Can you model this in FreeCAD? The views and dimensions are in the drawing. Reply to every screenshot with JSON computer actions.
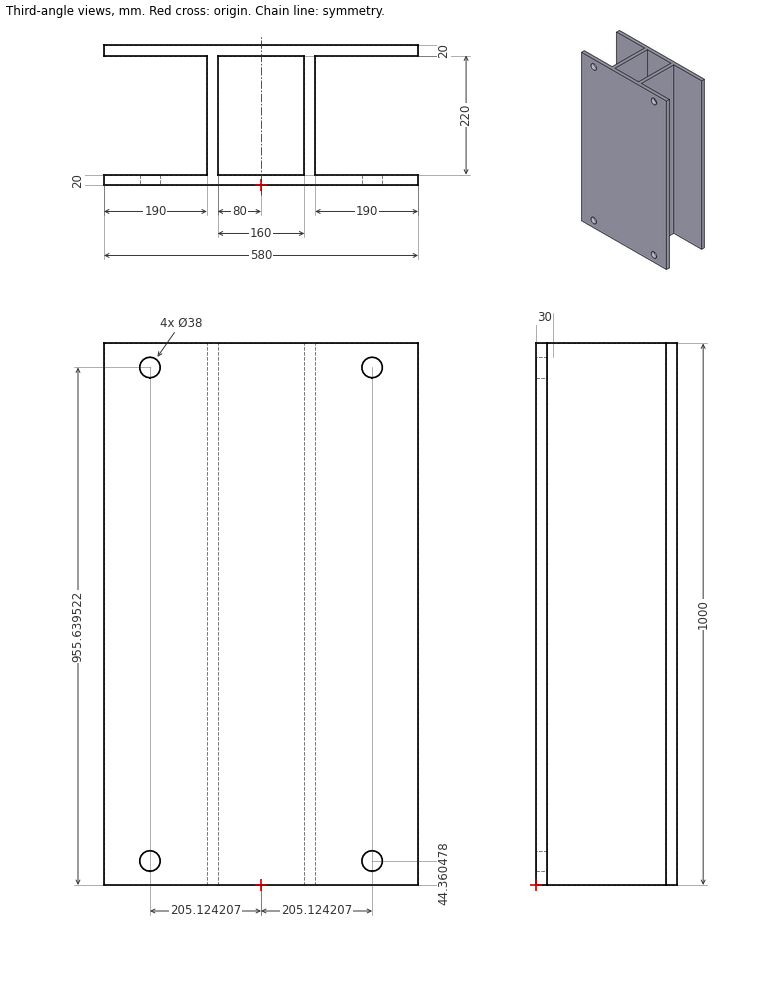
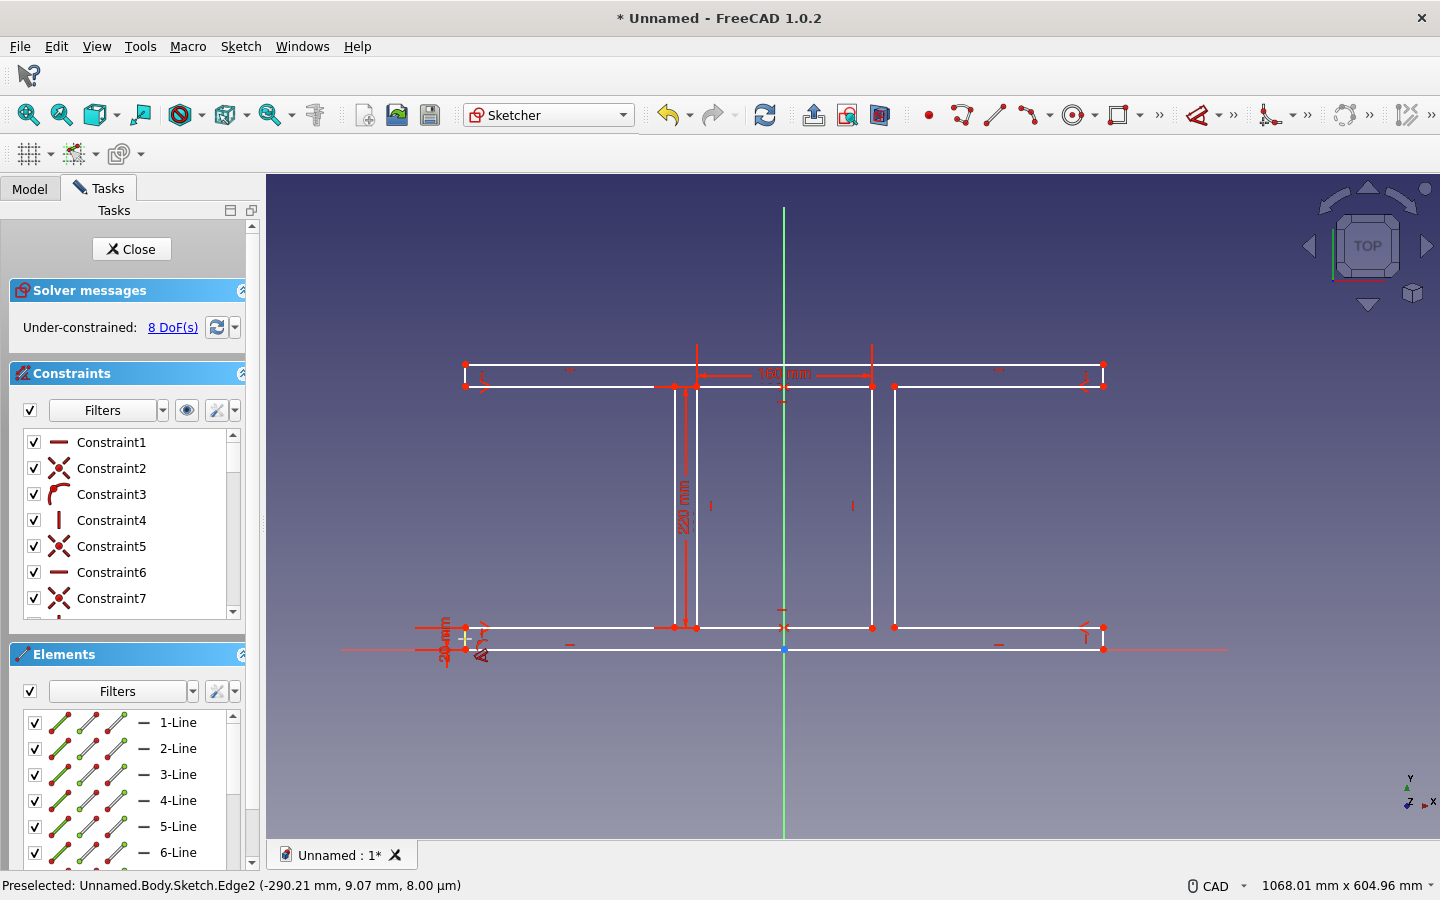
{"action": "scroll", "coordinate": [1103, 380], "scroll_direction": "up", "scroll_amount": 4}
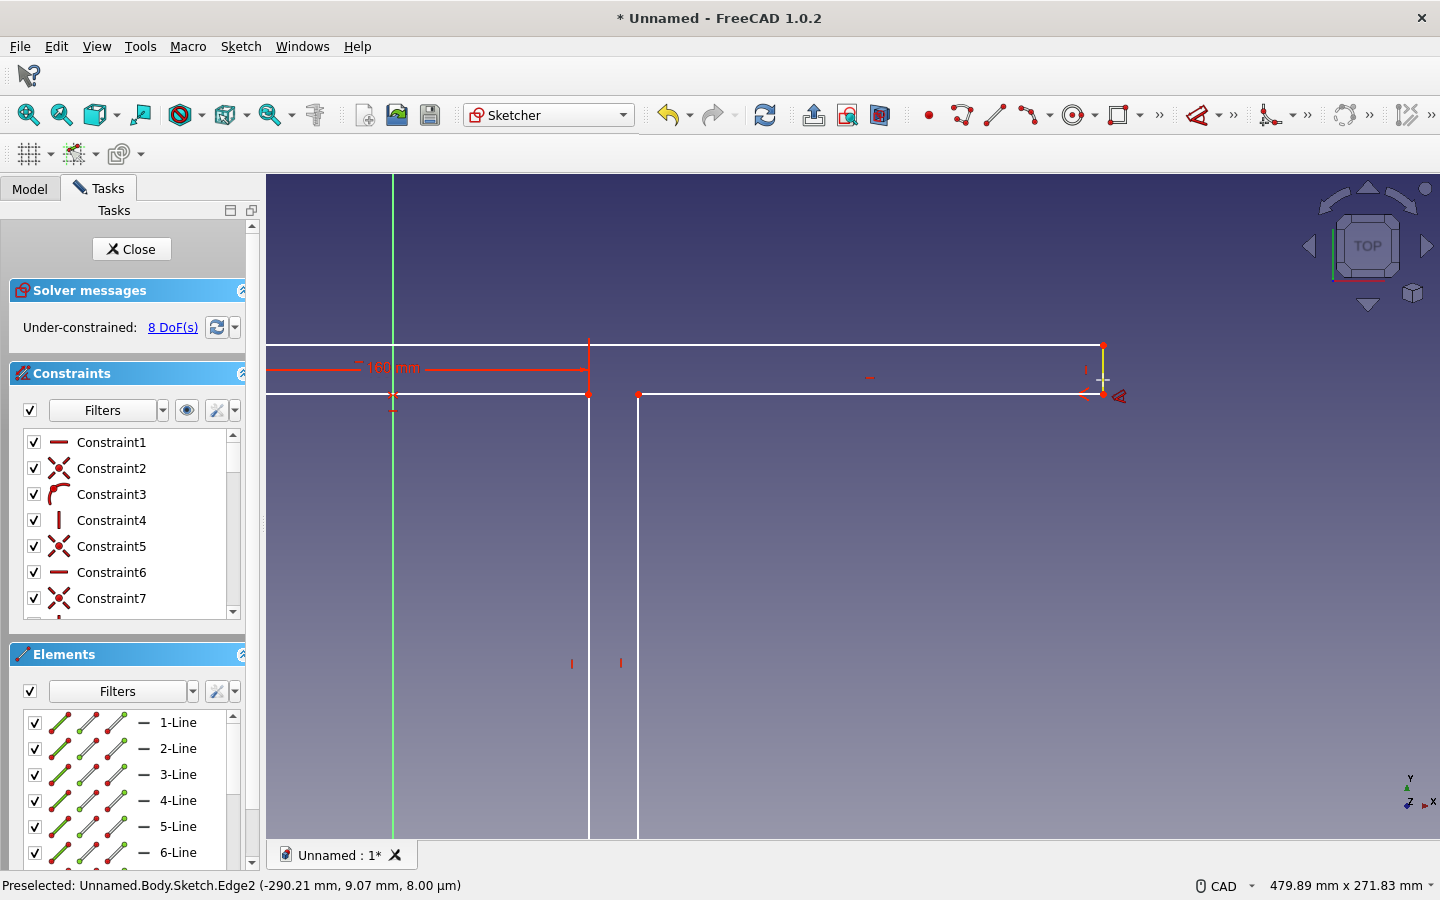
{"action": "left_click", "coordinate": [1103, 380]}
{"action": "left_click", "coordinate": [1137, 370]}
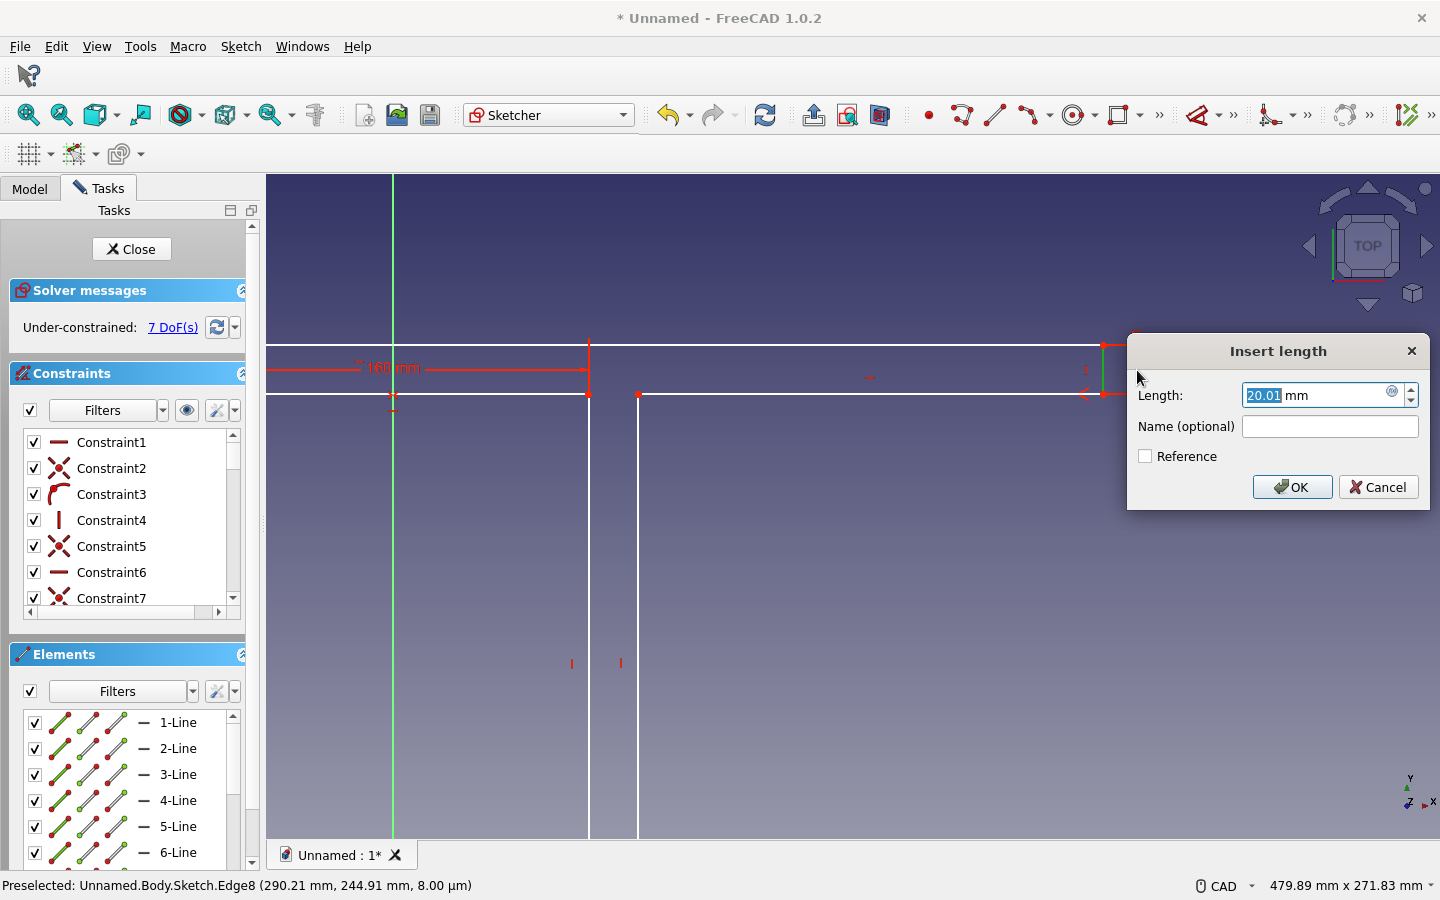
{"action": "type", "text": "20"}
{"action": "key", "text": "Return"}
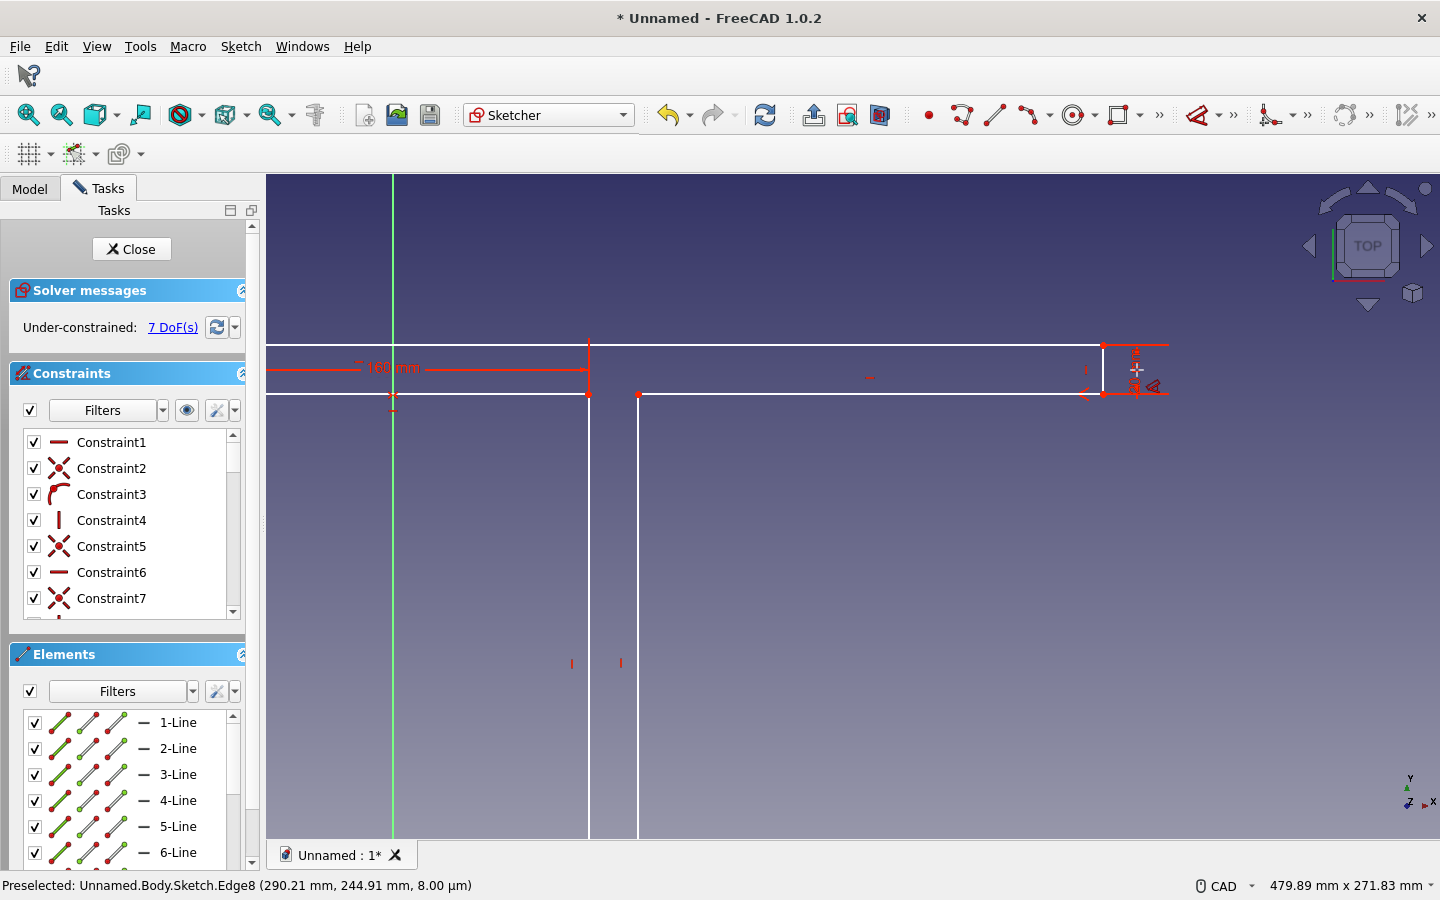
{"action": "scroll", "coordinate": [1104, 380], "scroll_direction": "down", "scroll_amount": 4}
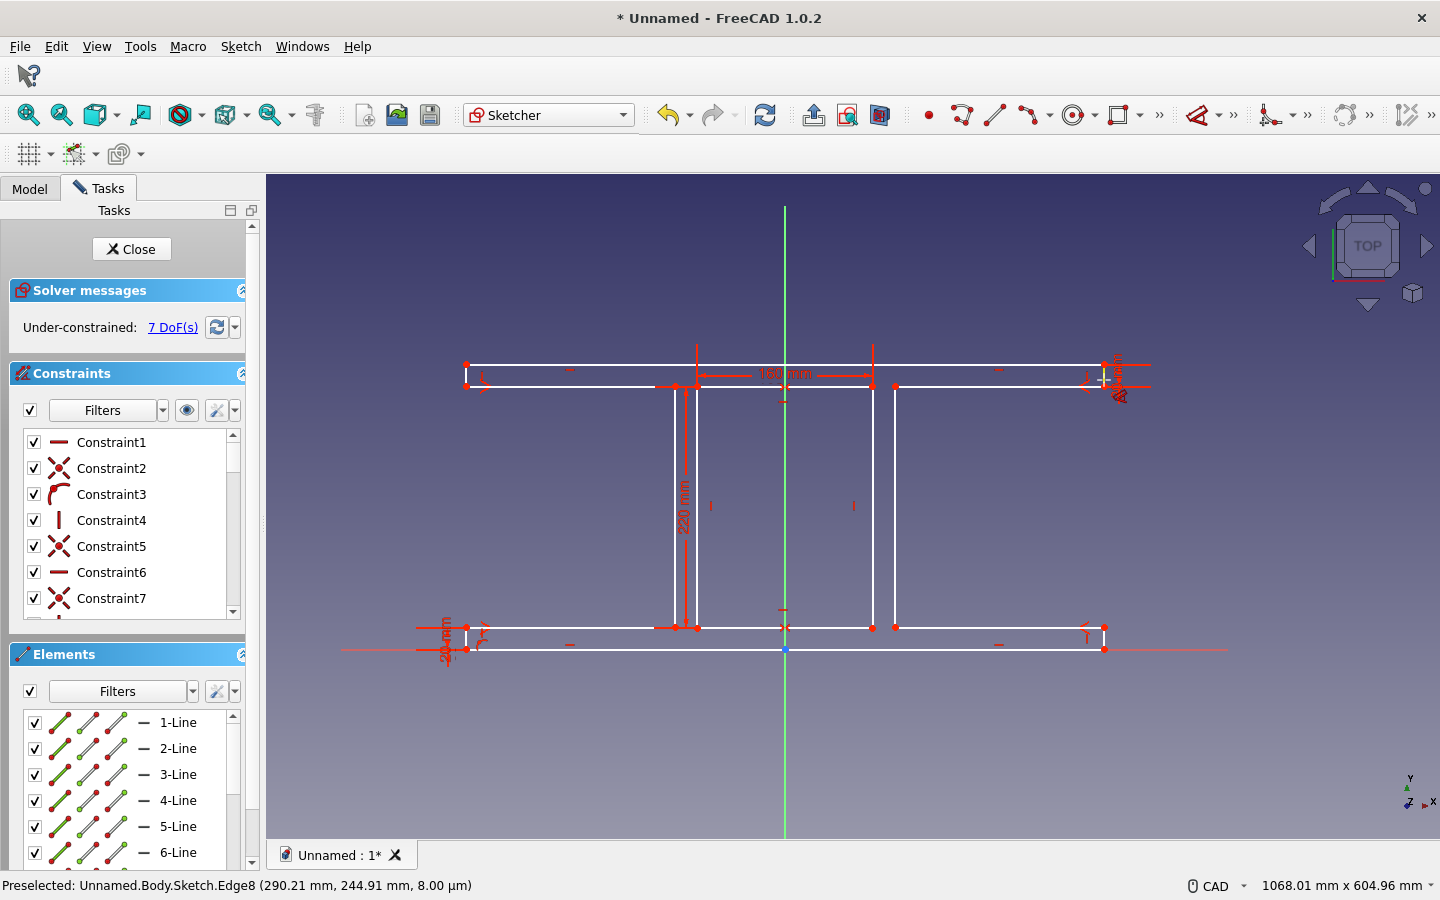
{"action": "left_click", "coordinate": [612, 628]}
{"action": "left_click", "coordinate": [571, 594]}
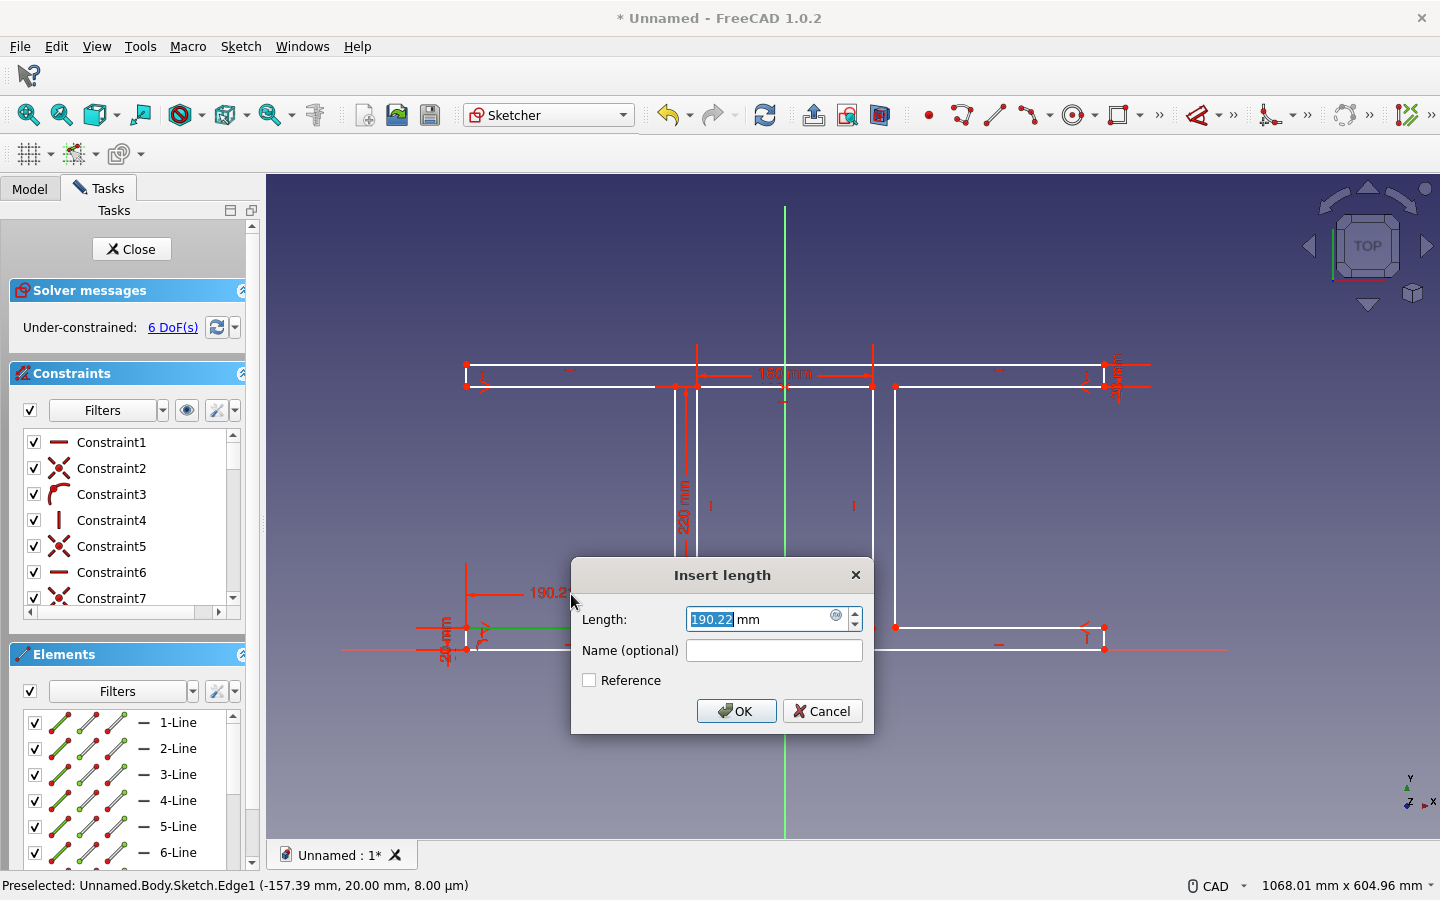
{"action": "type", "text": "190"}
{"action": "key", "text": "Return"}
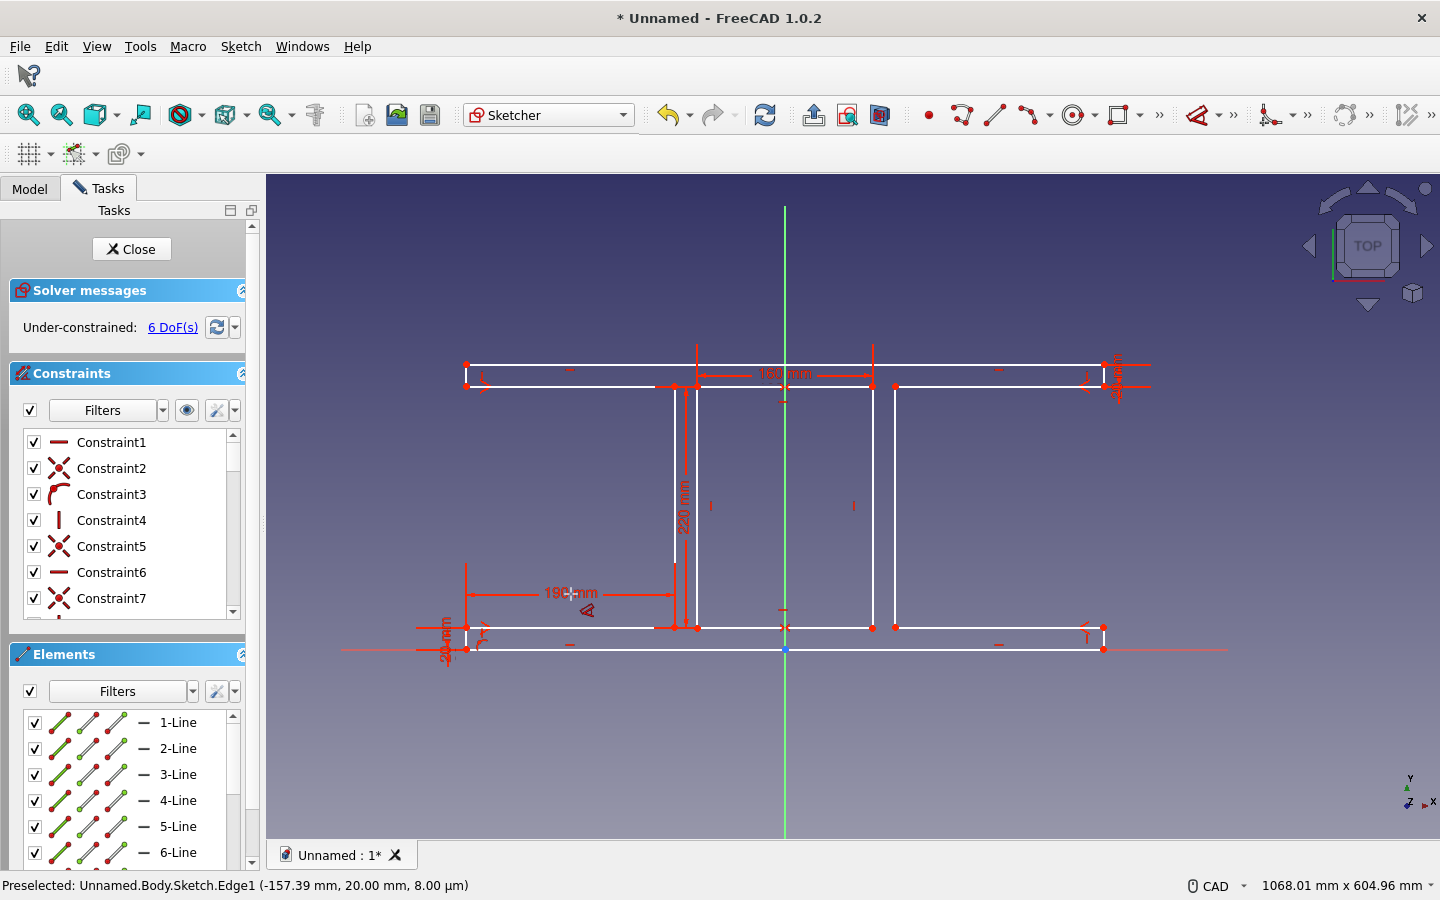
{"action": "left_click", "coordinate": [657, 650]}
{"action": "left_click", "coordinate": [638, 684]}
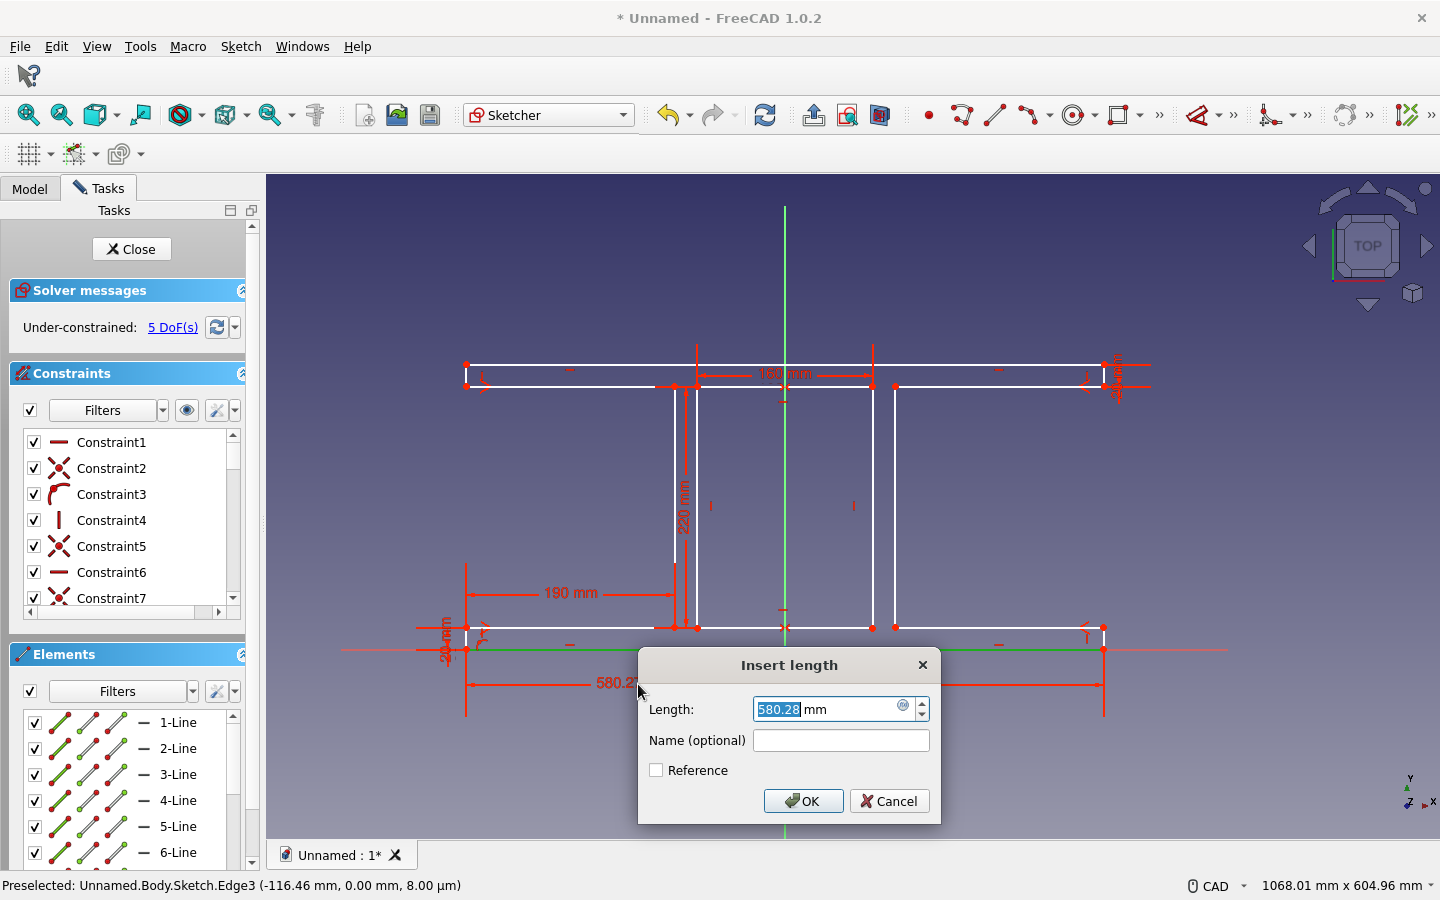
{"action": "type", "text": "580"}
{"action": "key", "text": "Return"}